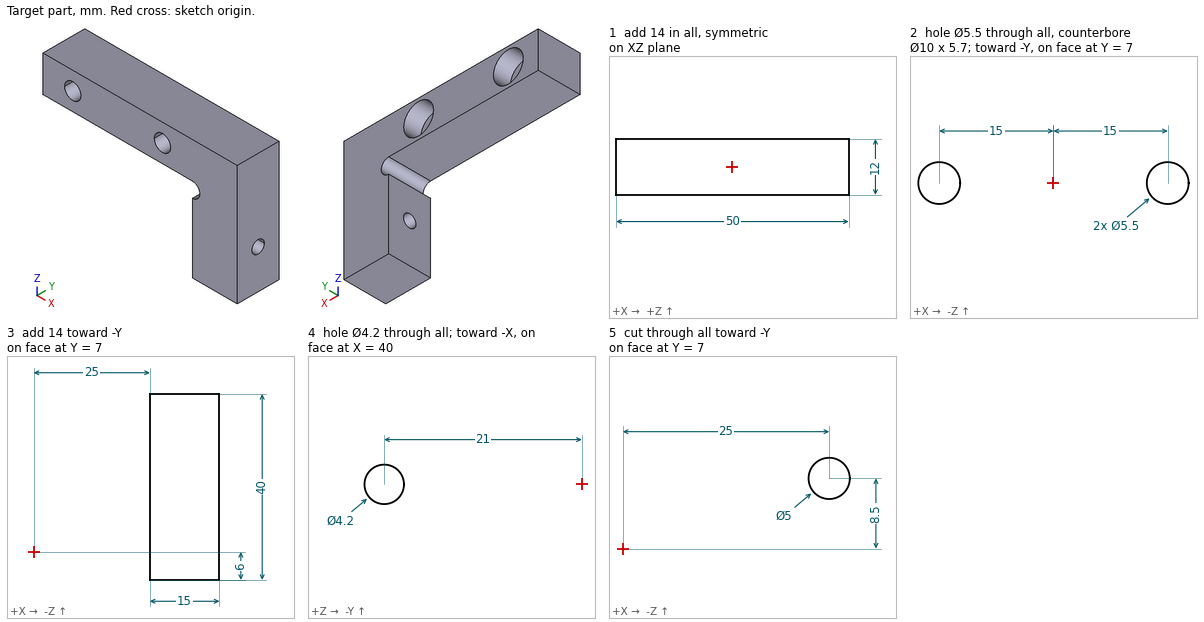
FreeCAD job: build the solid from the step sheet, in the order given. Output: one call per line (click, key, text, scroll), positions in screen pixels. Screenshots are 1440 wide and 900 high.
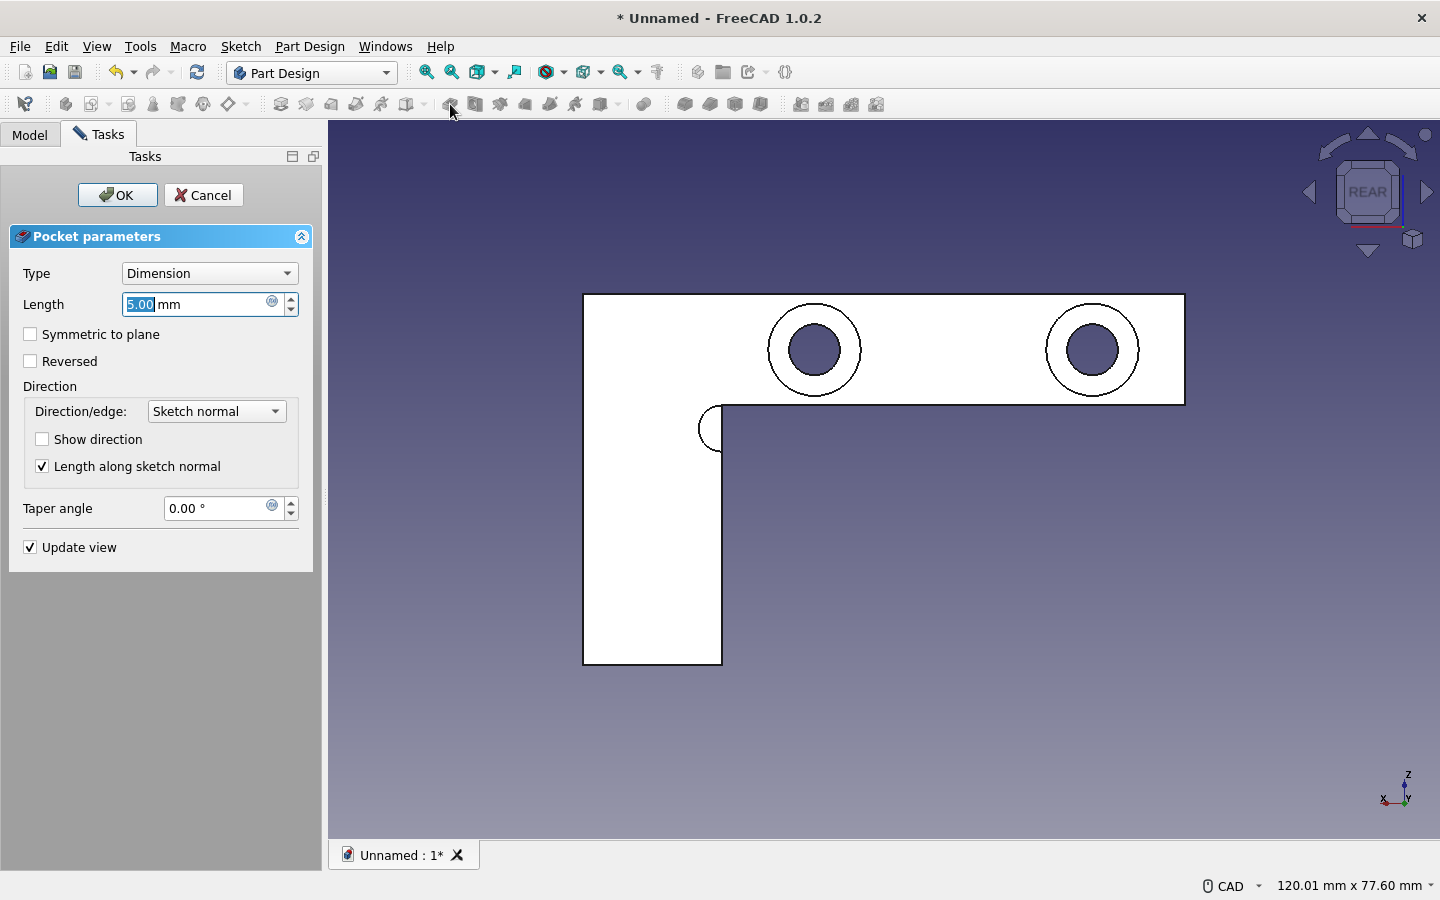
click(210, 274)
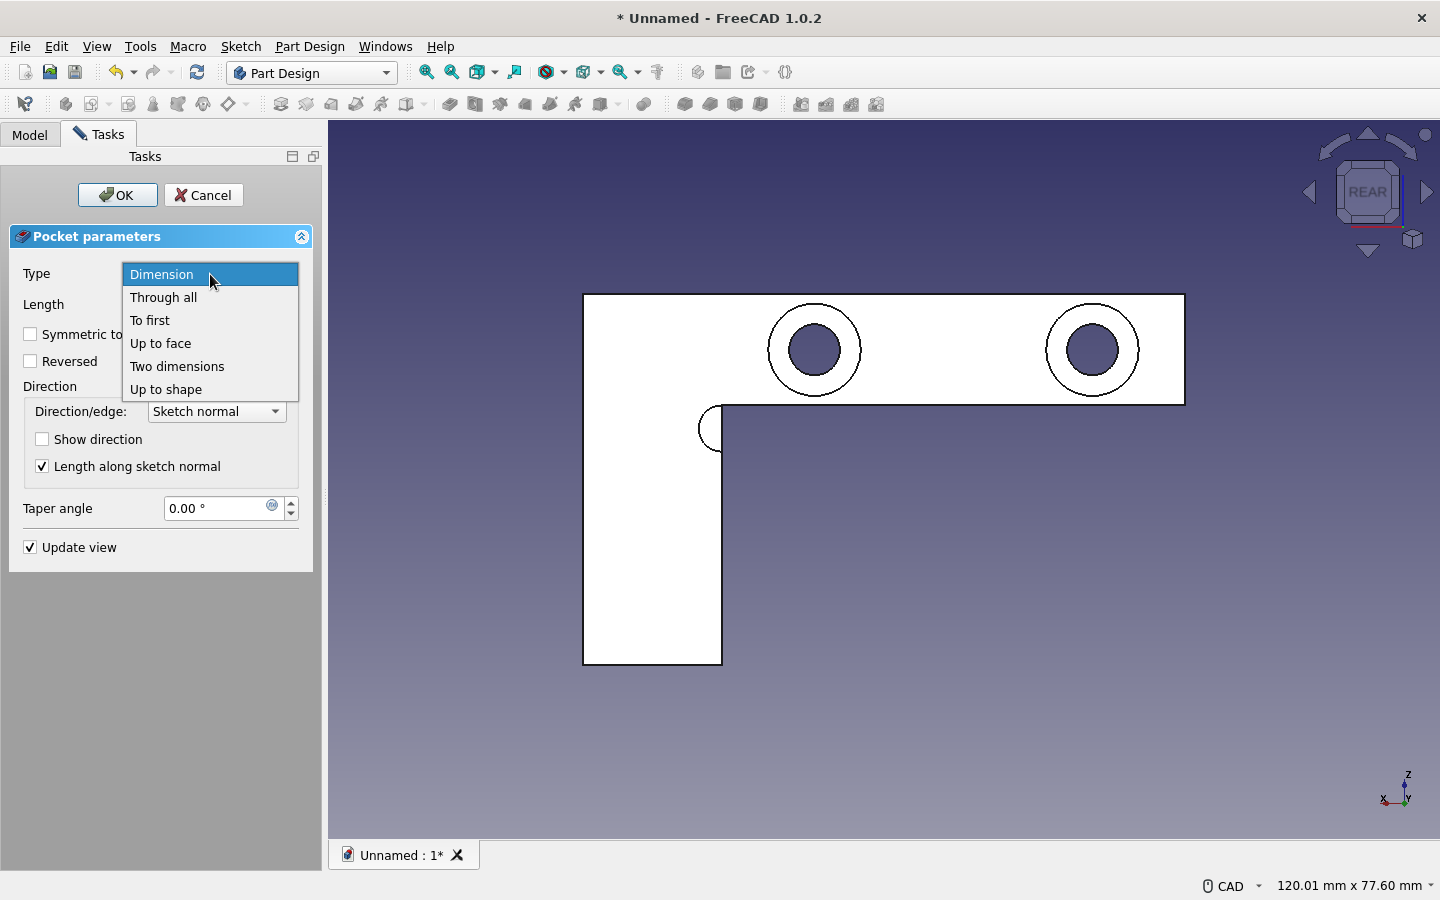
click(208, 298)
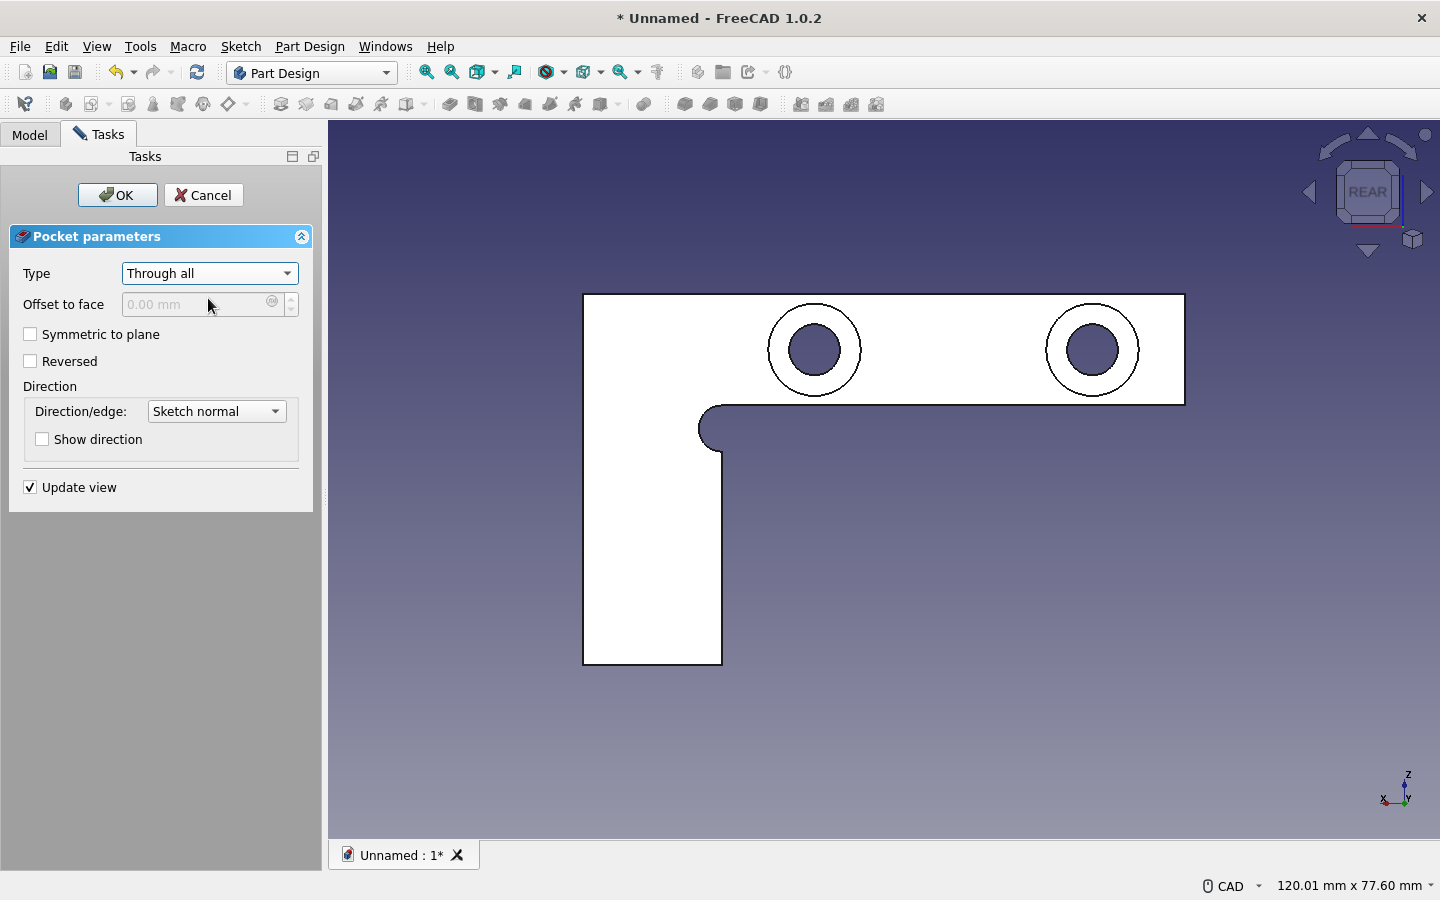
click(118, 195)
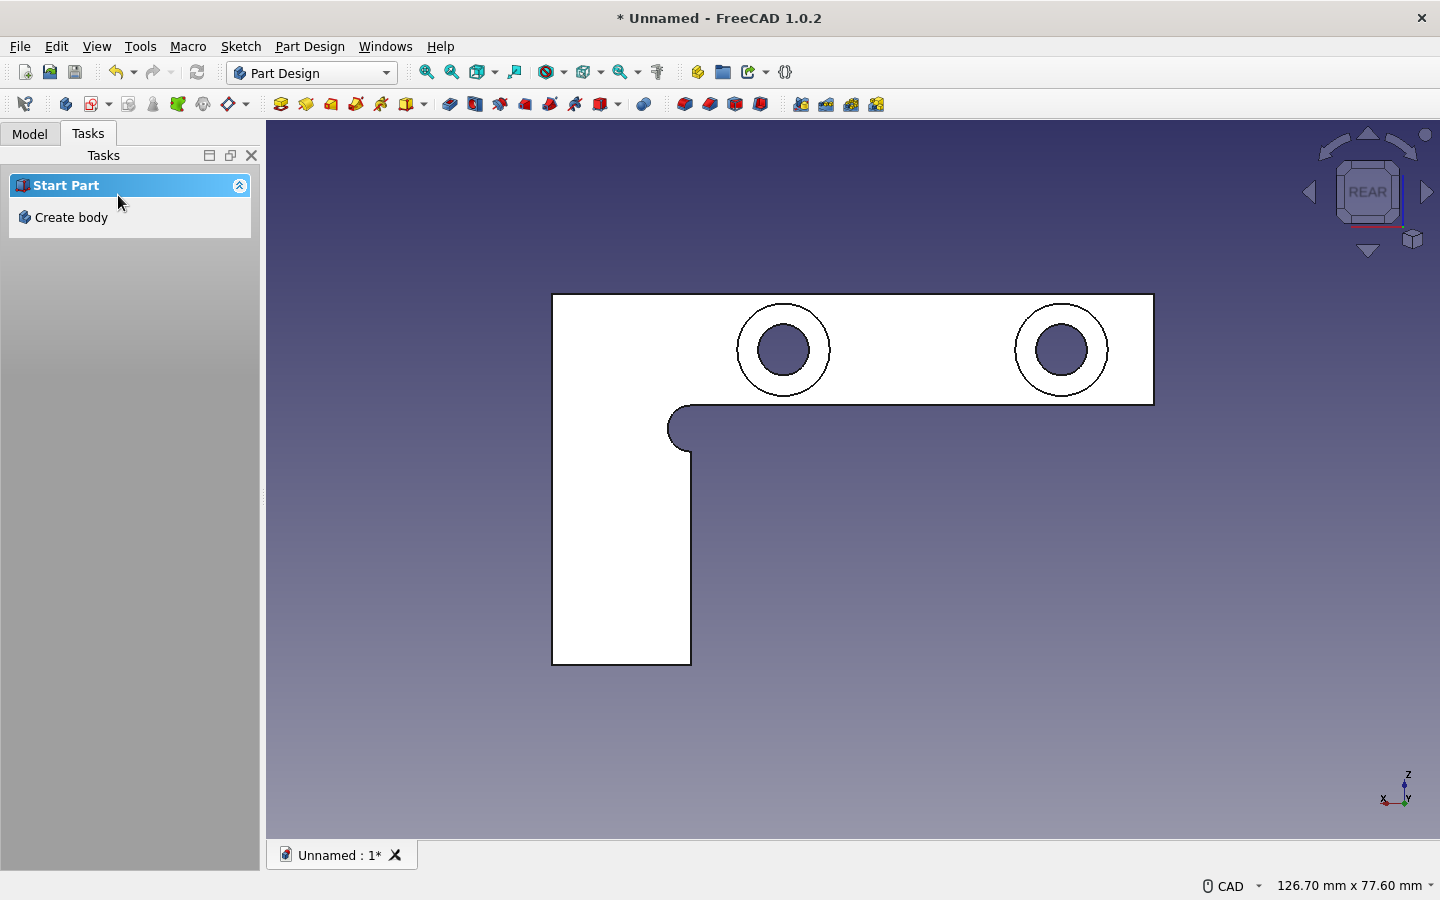
key(0)